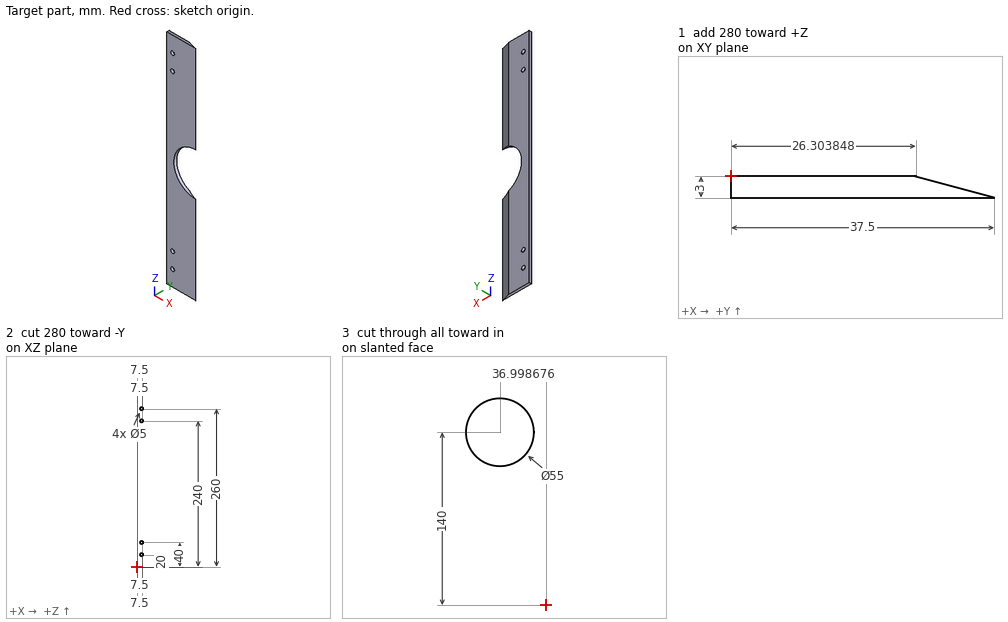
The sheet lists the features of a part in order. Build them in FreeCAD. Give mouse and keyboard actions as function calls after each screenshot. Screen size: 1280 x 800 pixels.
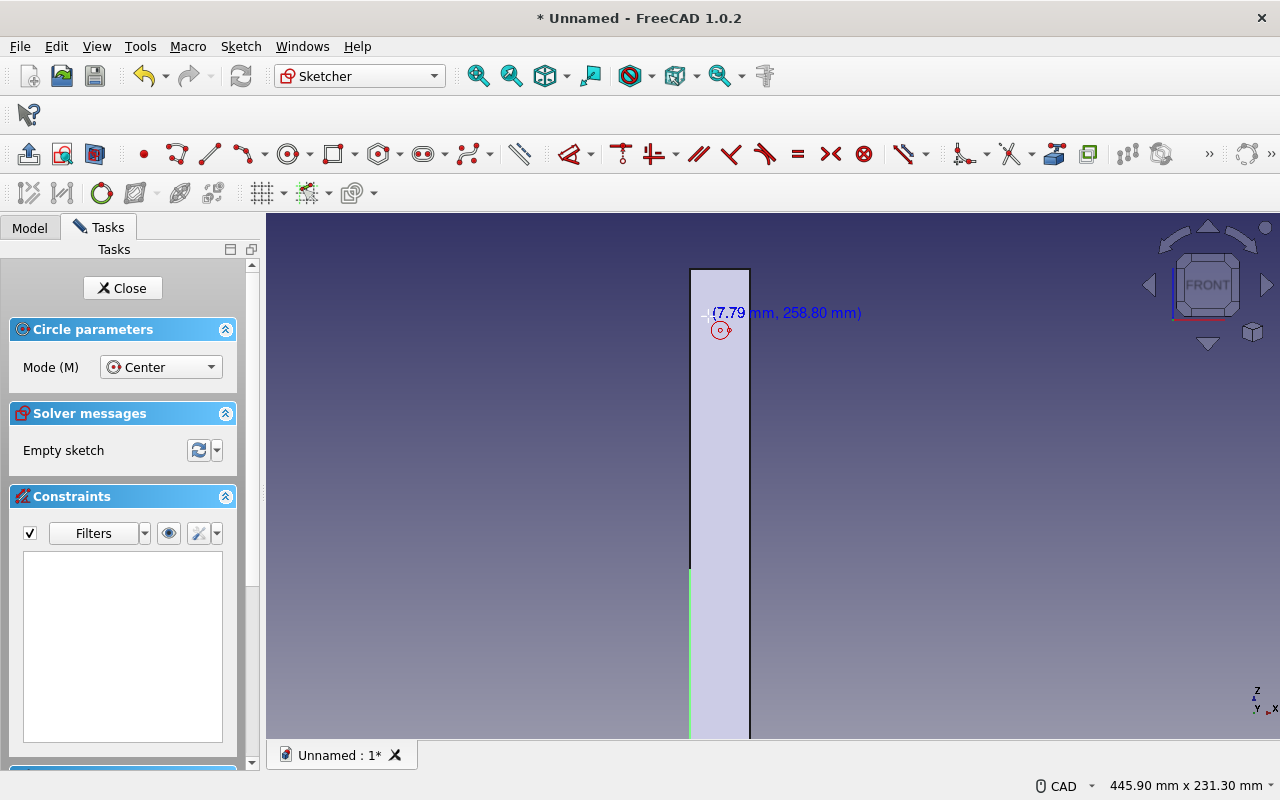
click(707, 315)
move(711, 311)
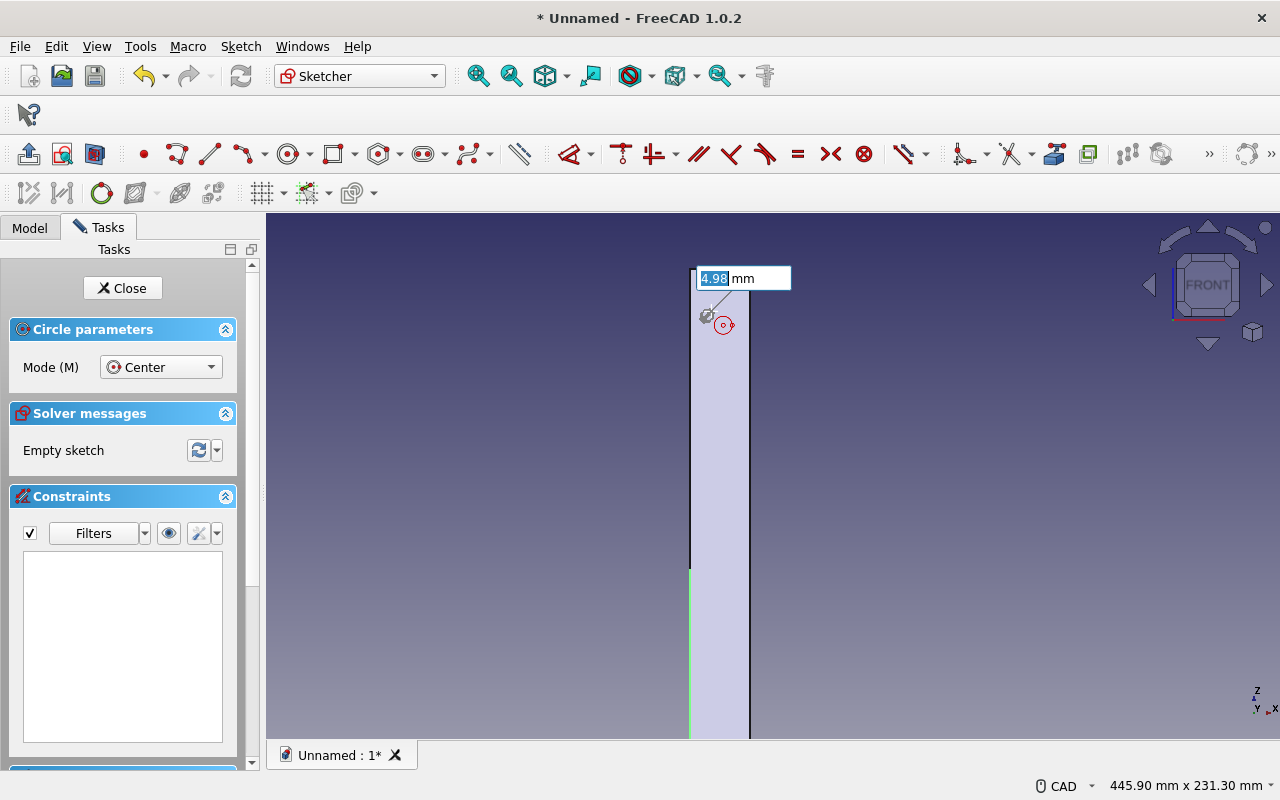
text(5)
key(Return)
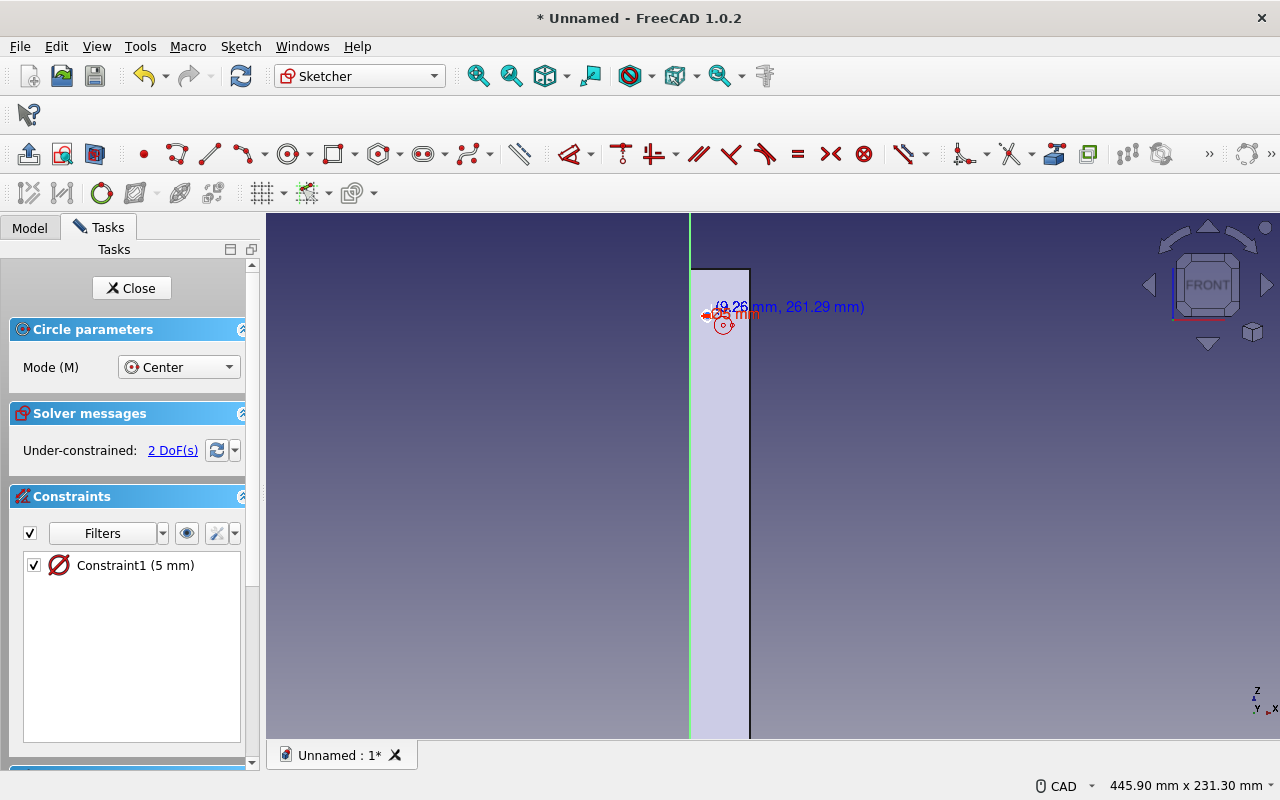
scroll(707, 360, up, 7)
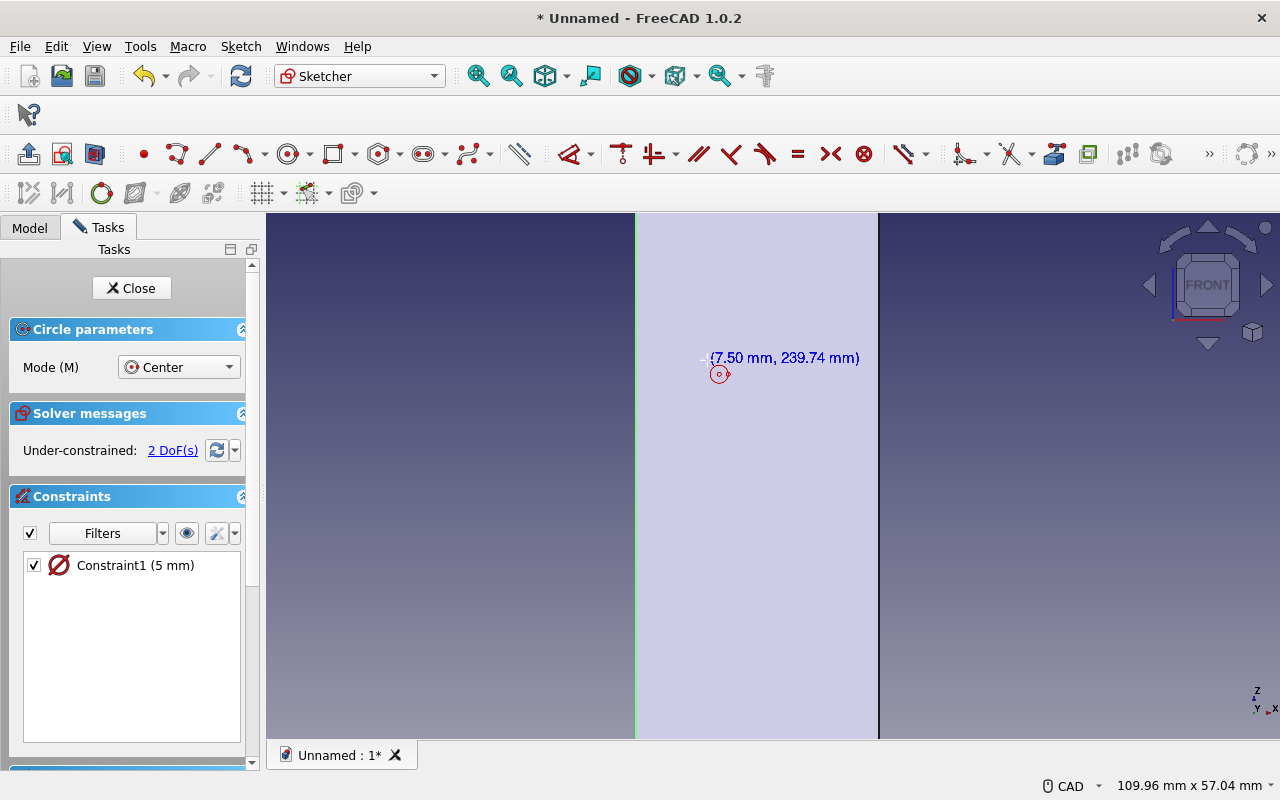
scroll(708, 337, down, 10)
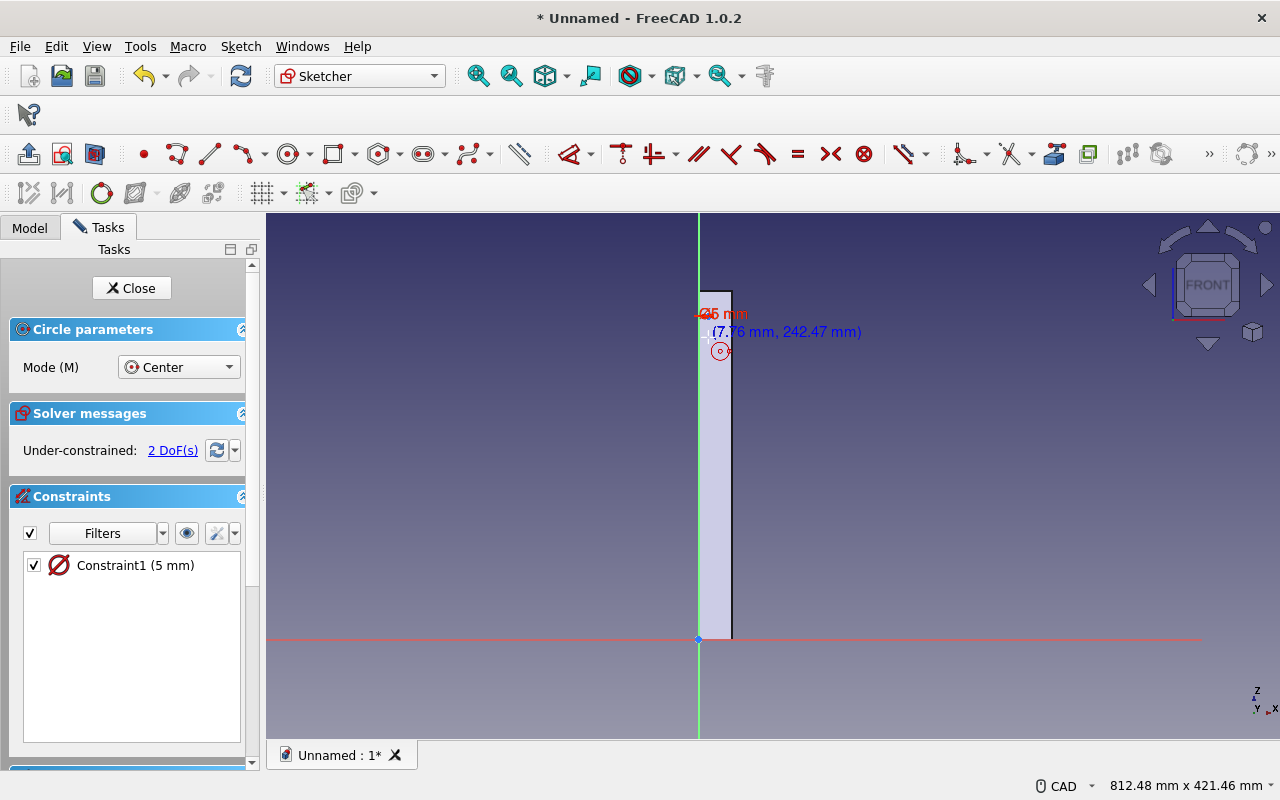
scroll(708, 340, up, 3)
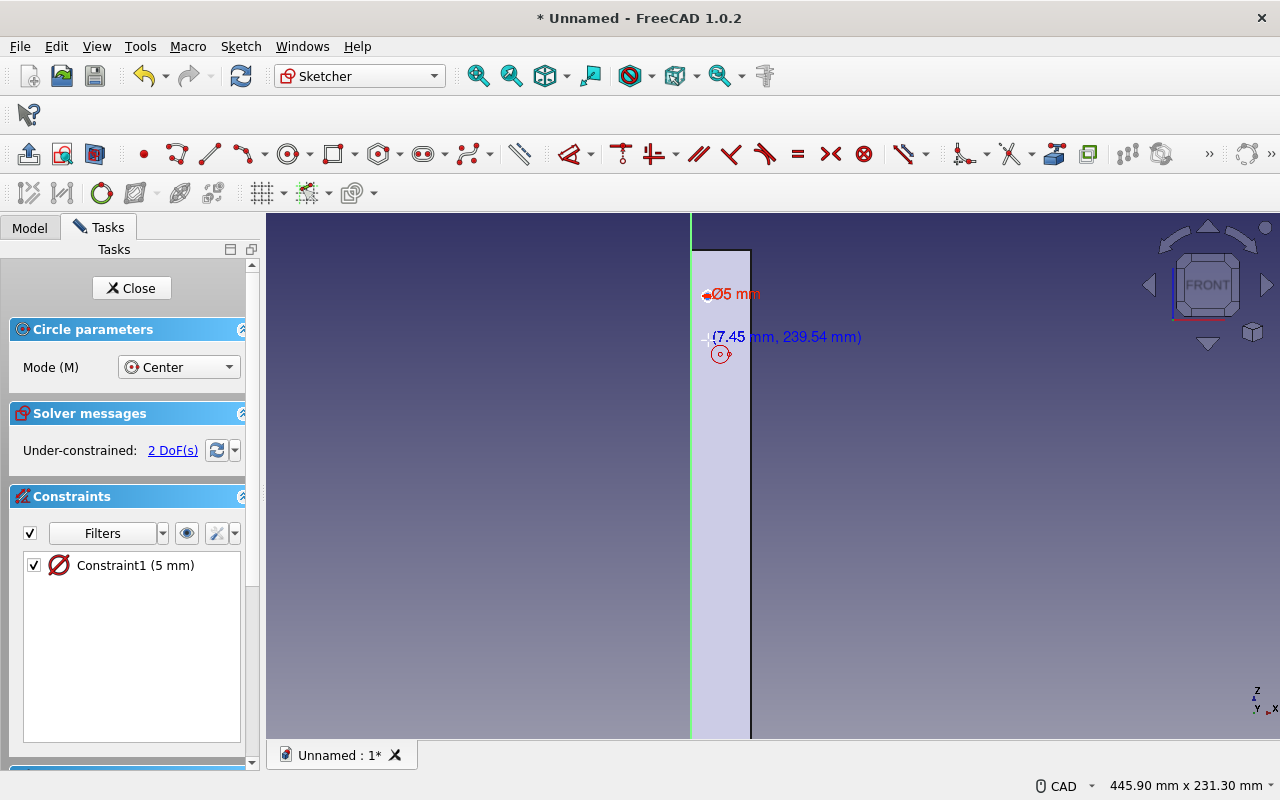
click(708, 341)
move(712, 337)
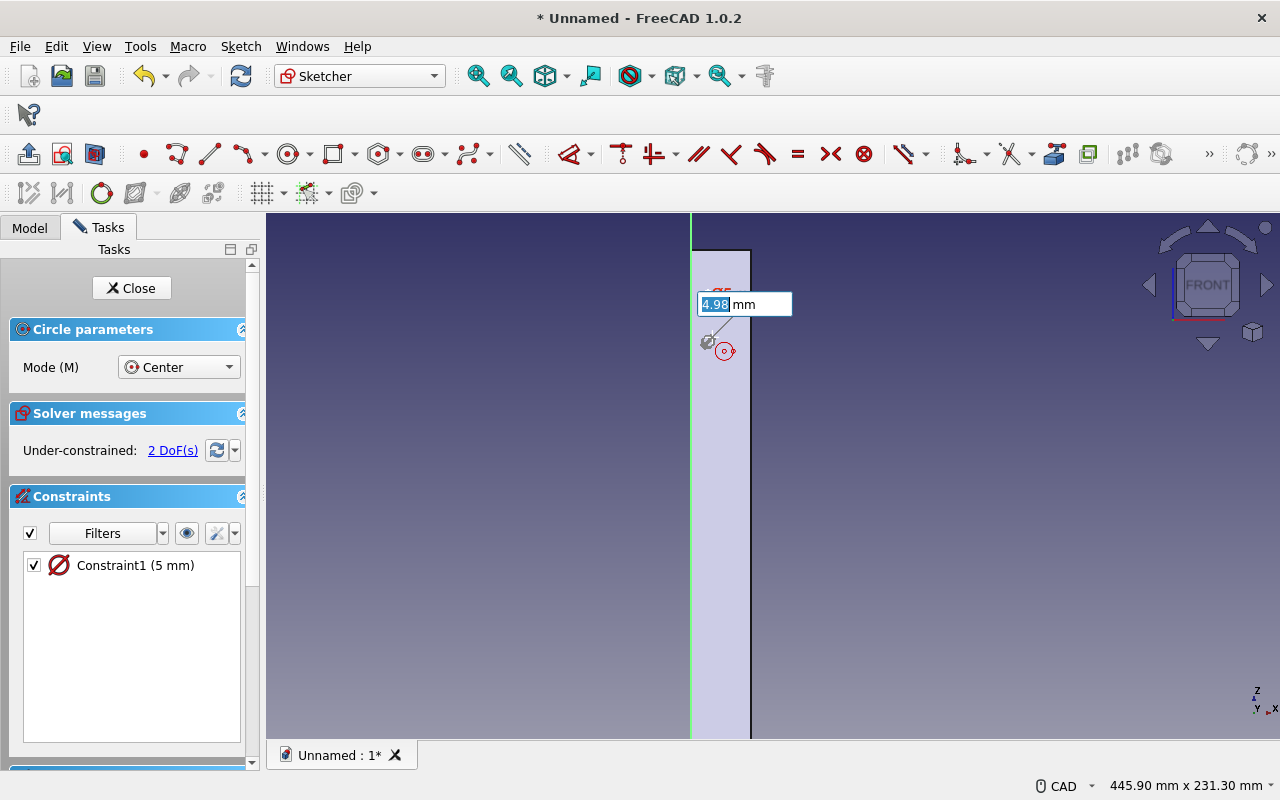
text(5)
key(Return)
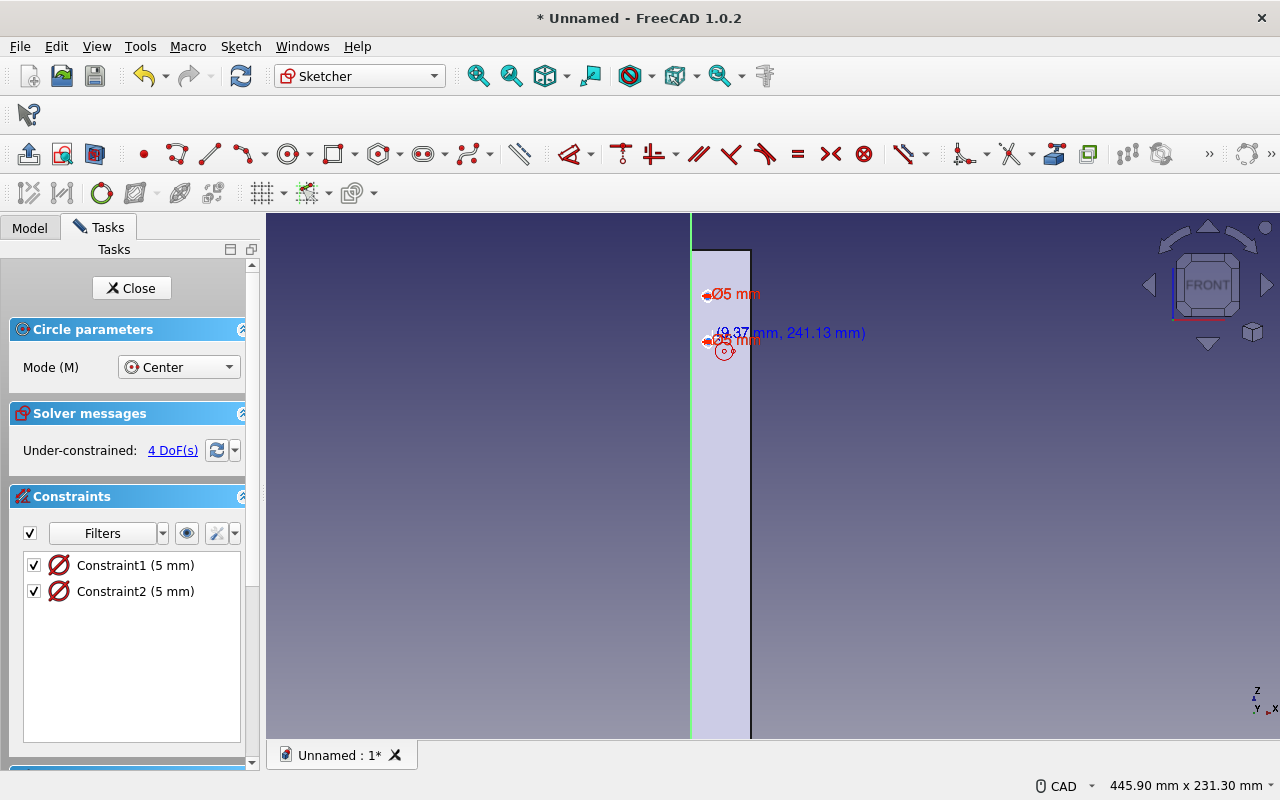
scroll(707, 340, down, 3)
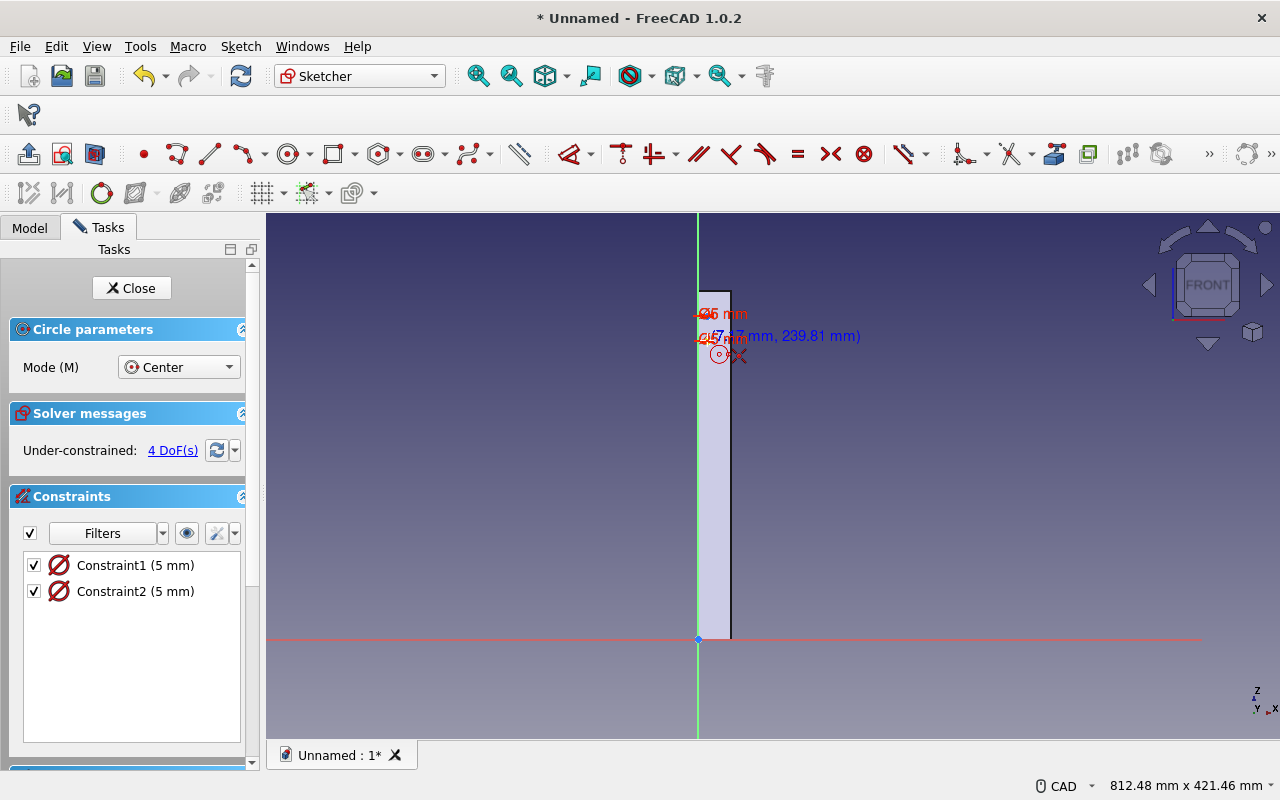
scroll(708, 615, up, 10)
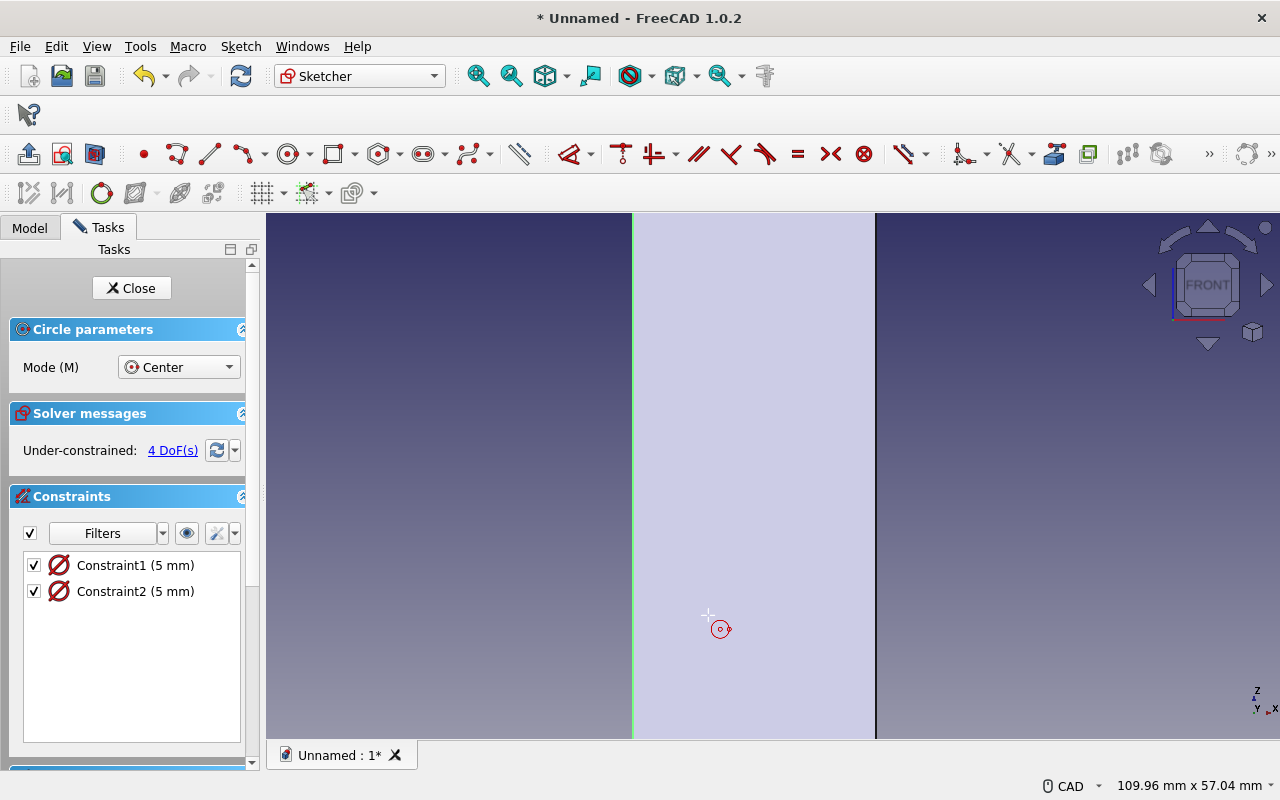
scroll(708, 616, down, 10)